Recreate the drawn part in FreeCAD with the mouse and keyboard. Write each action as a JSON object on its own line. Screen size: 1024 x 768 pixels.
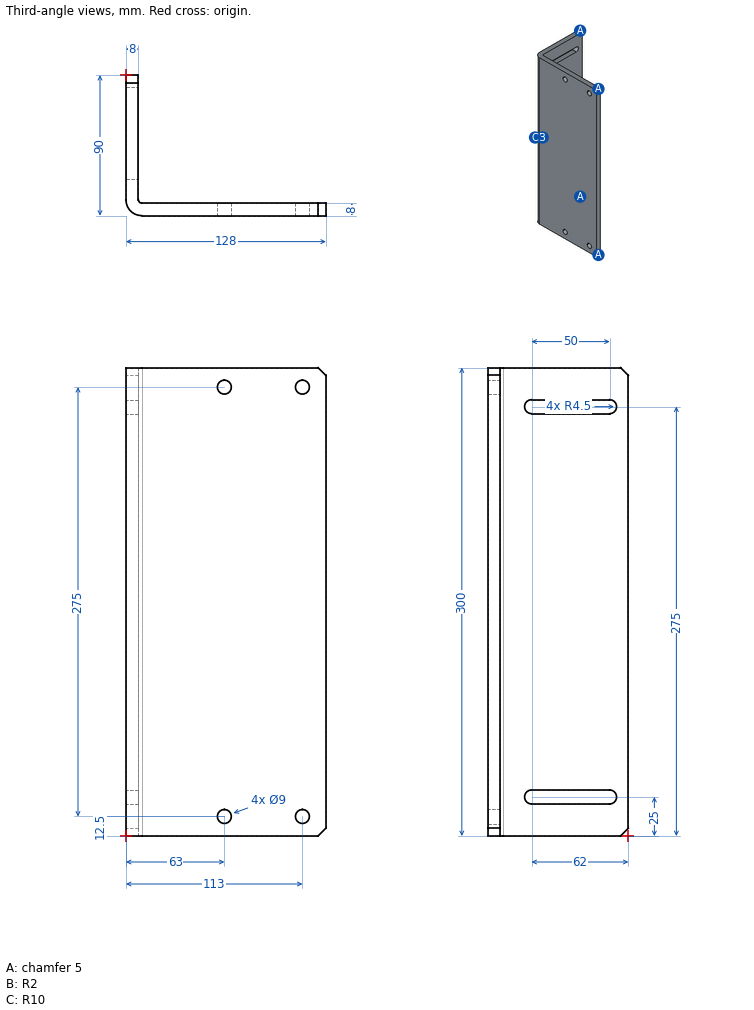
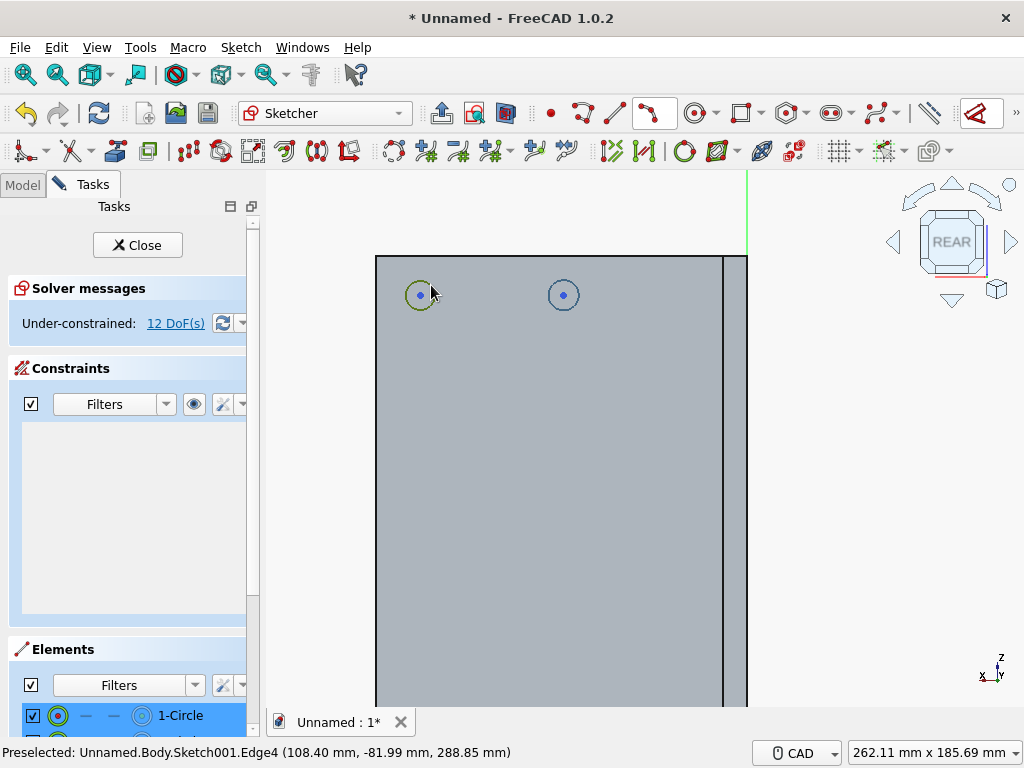
{"action": "key", "text": "e"}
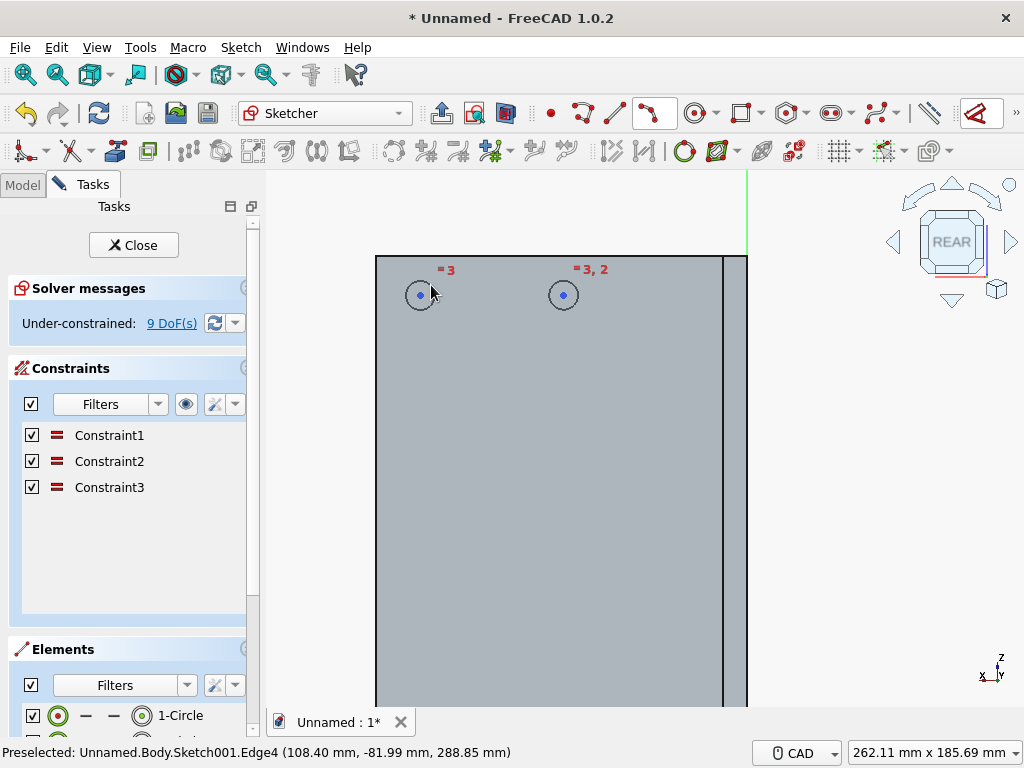
{"action": "scroll", "coordinate": [576, 285], "scroll_direction": "down", "scroll_amount": 5}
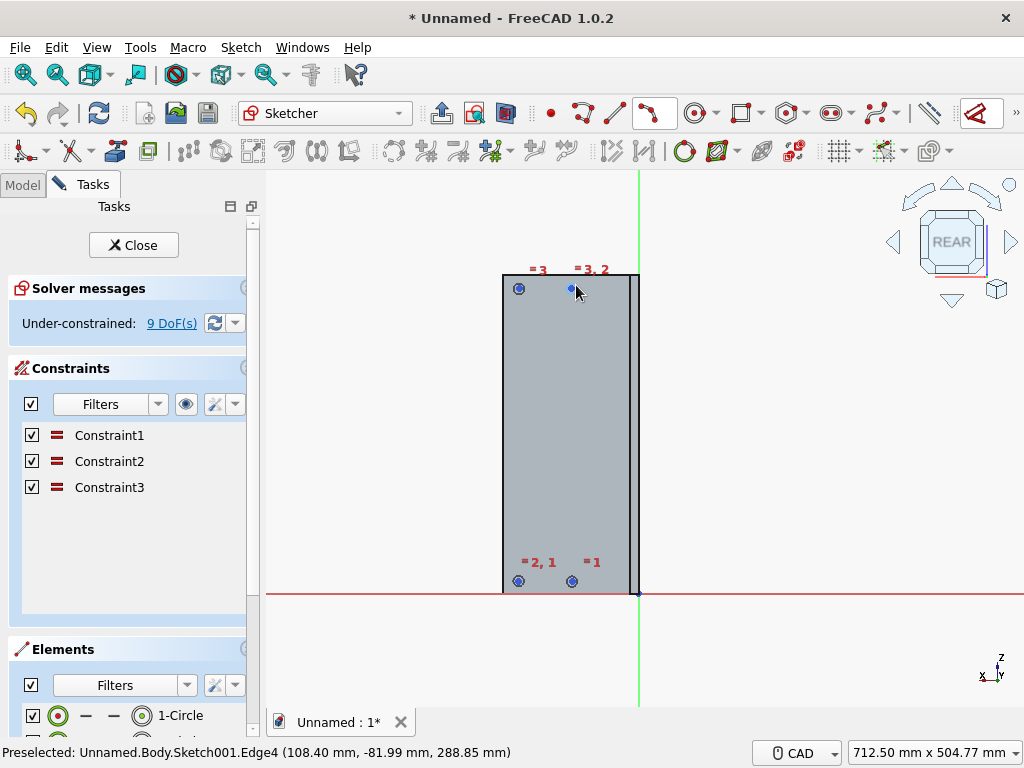
{"action": "left_click", "coordinate": [572, 582]}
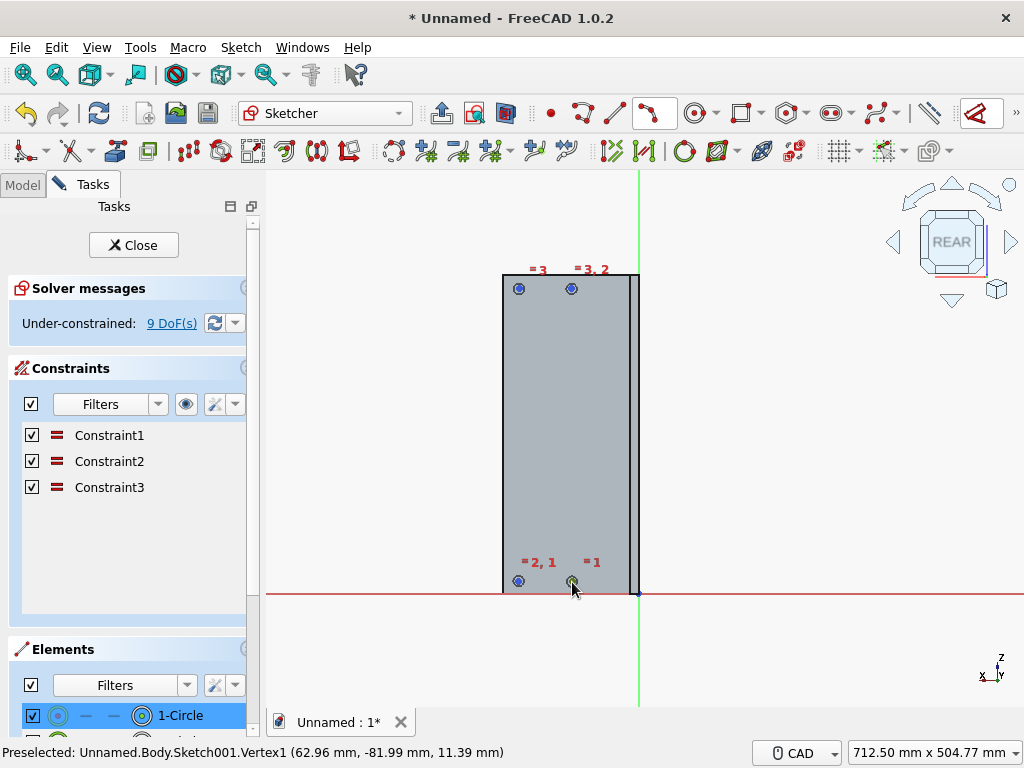
{"action": "left_click", "coordinate": [519, 581]}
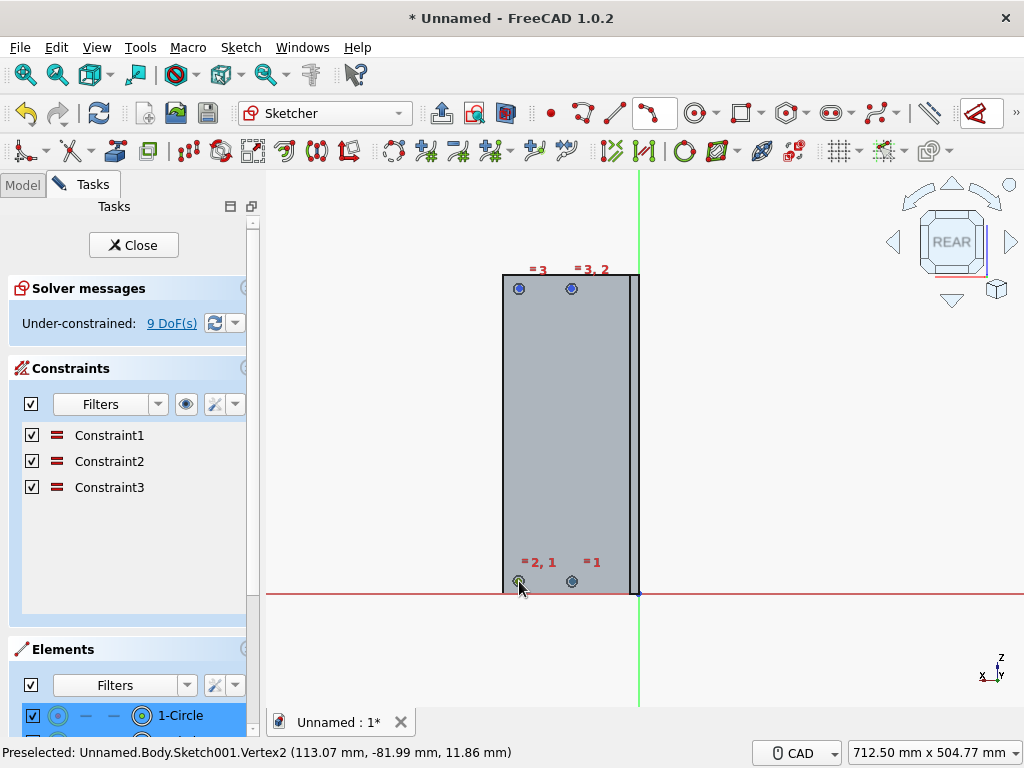
{"action": "key", "text": "h"}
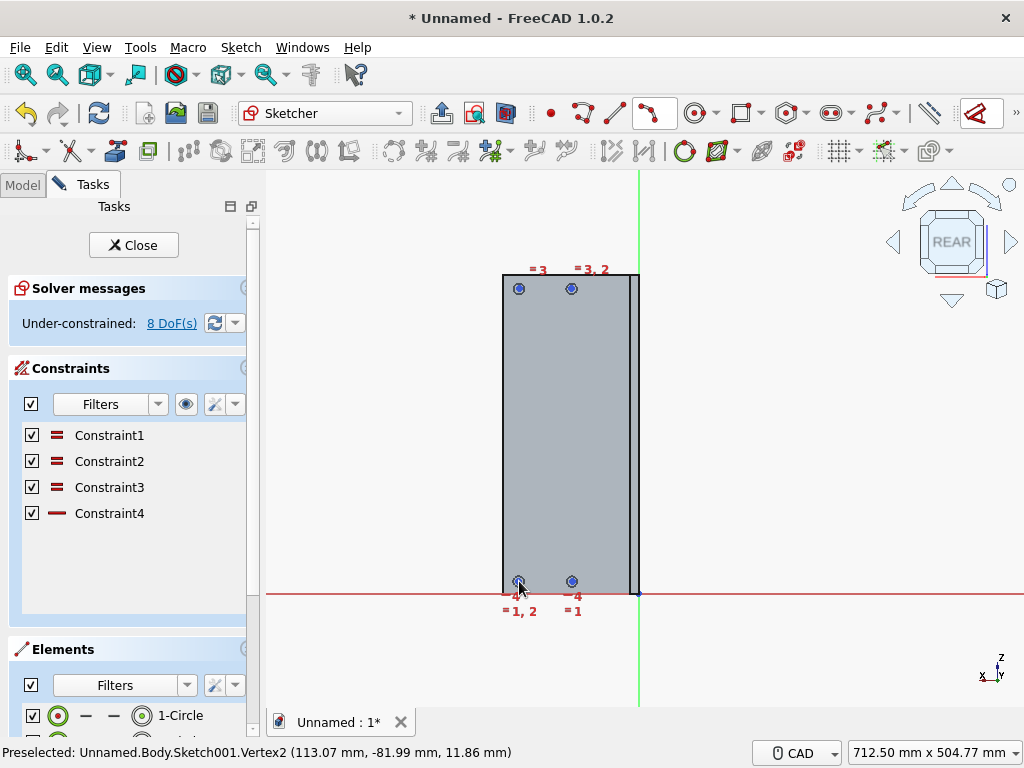
{"action": "left_click", "coordinate": [572, 582]}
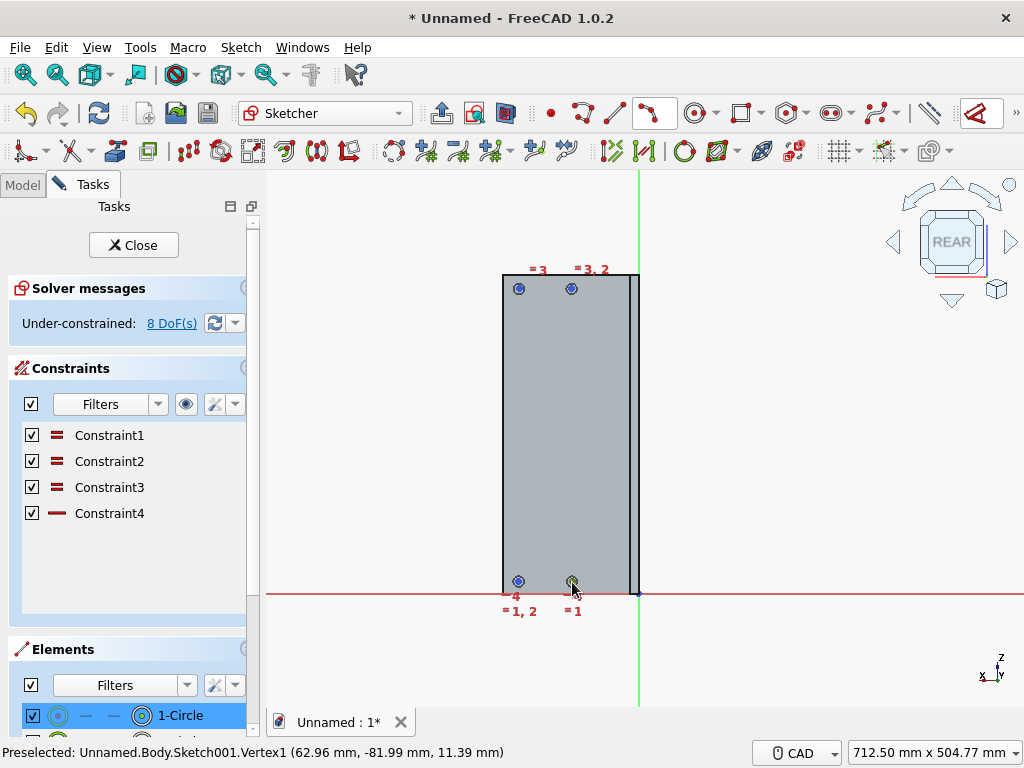
{"action": "left_click", "coordinate": [572, 289]}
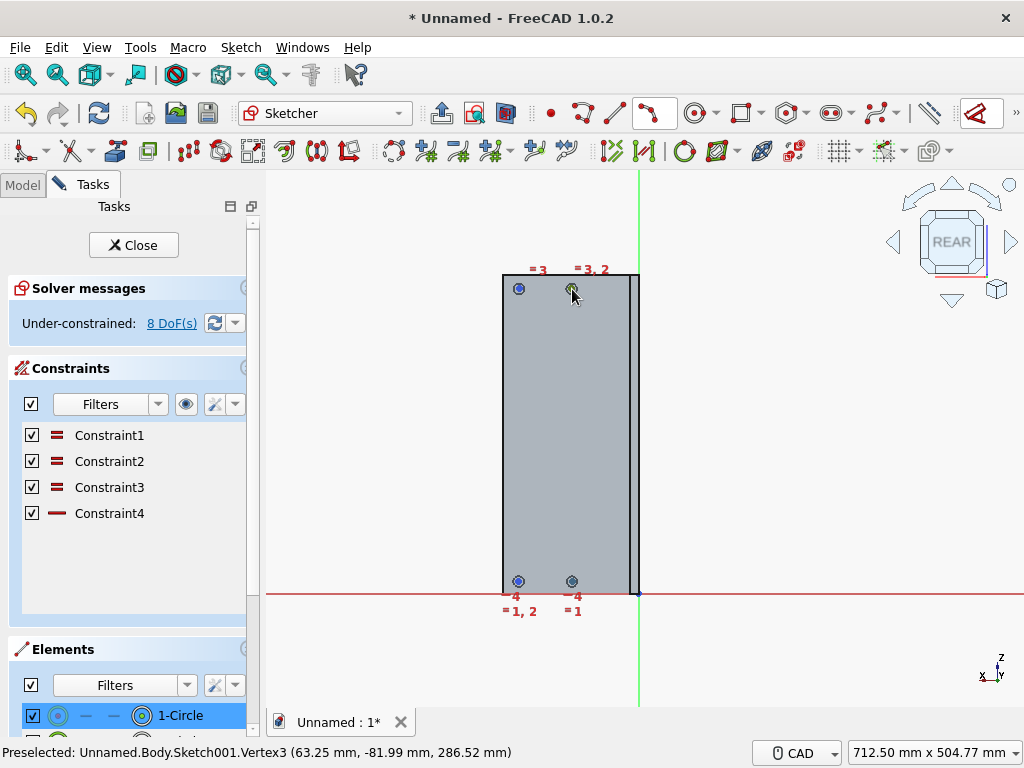
{"action": "key", "text": "v"}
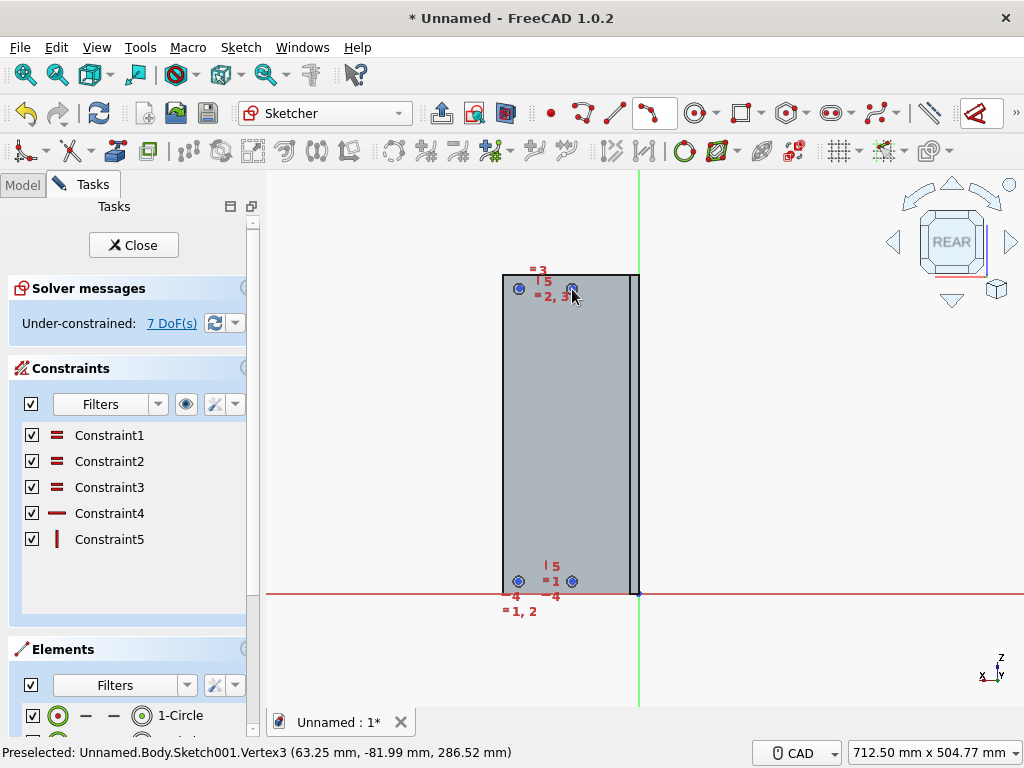
{"action": "left_click", "coordinate": [519, 582]}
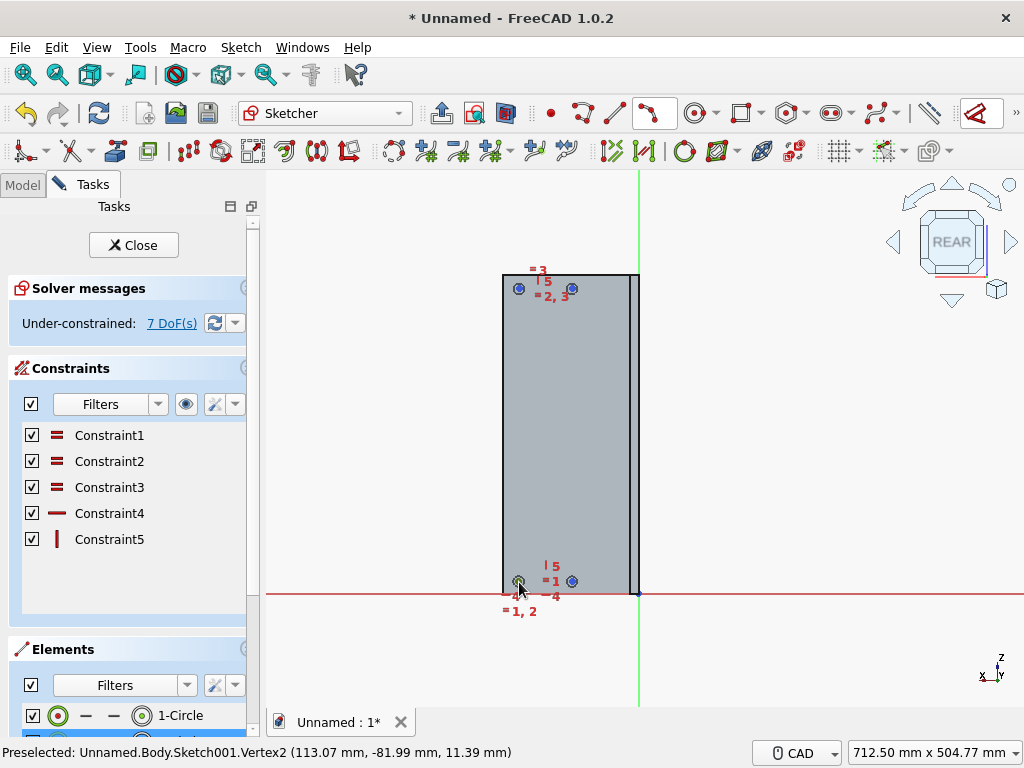
{"action": "left_click", "coordinate": [519, 289]}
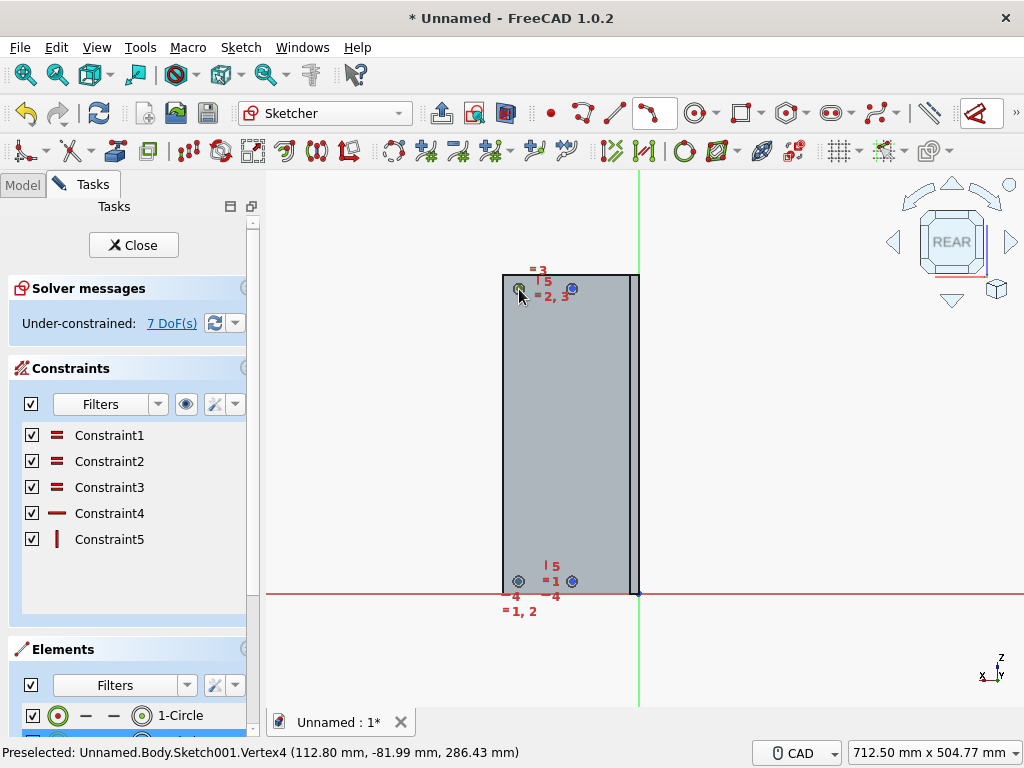
{"action": "key", "text": "v"}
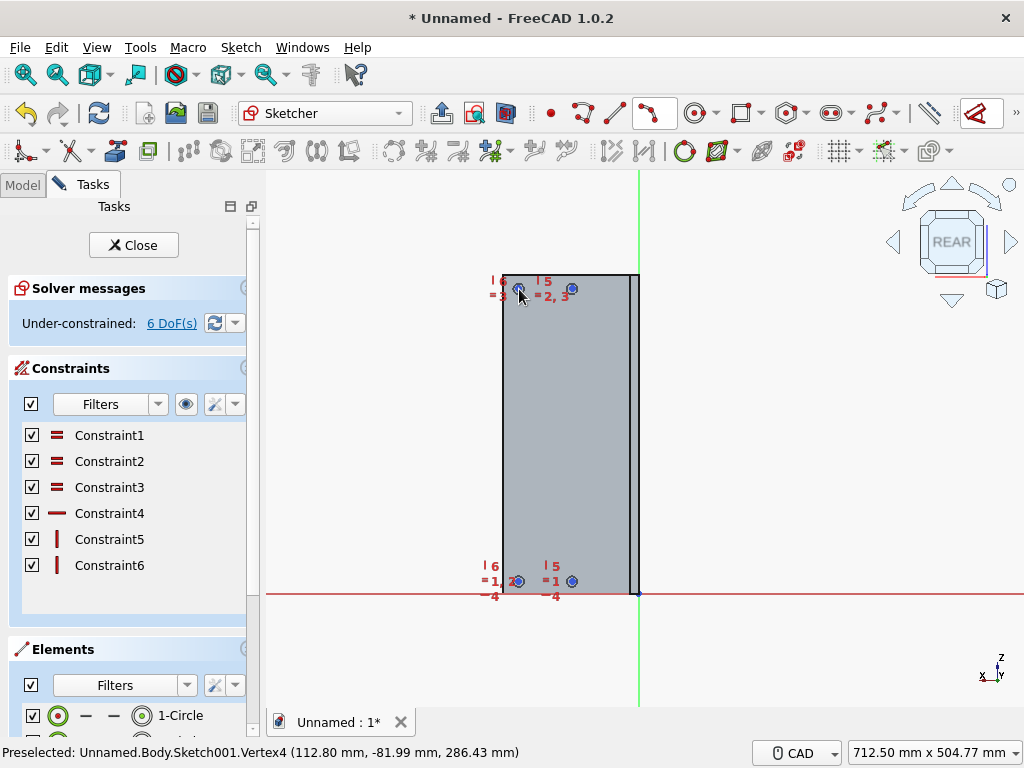
{"action": "left_click", "coordinate": [572, 289]}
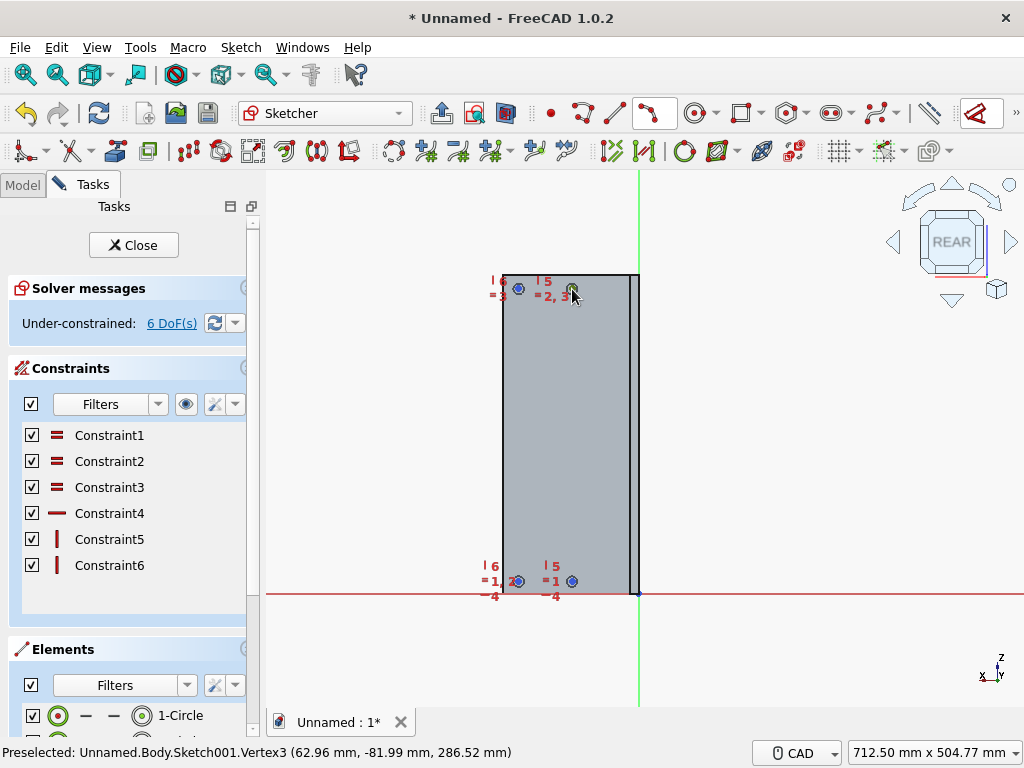
{"action": "left_click", "coordinate": [519, 289]}